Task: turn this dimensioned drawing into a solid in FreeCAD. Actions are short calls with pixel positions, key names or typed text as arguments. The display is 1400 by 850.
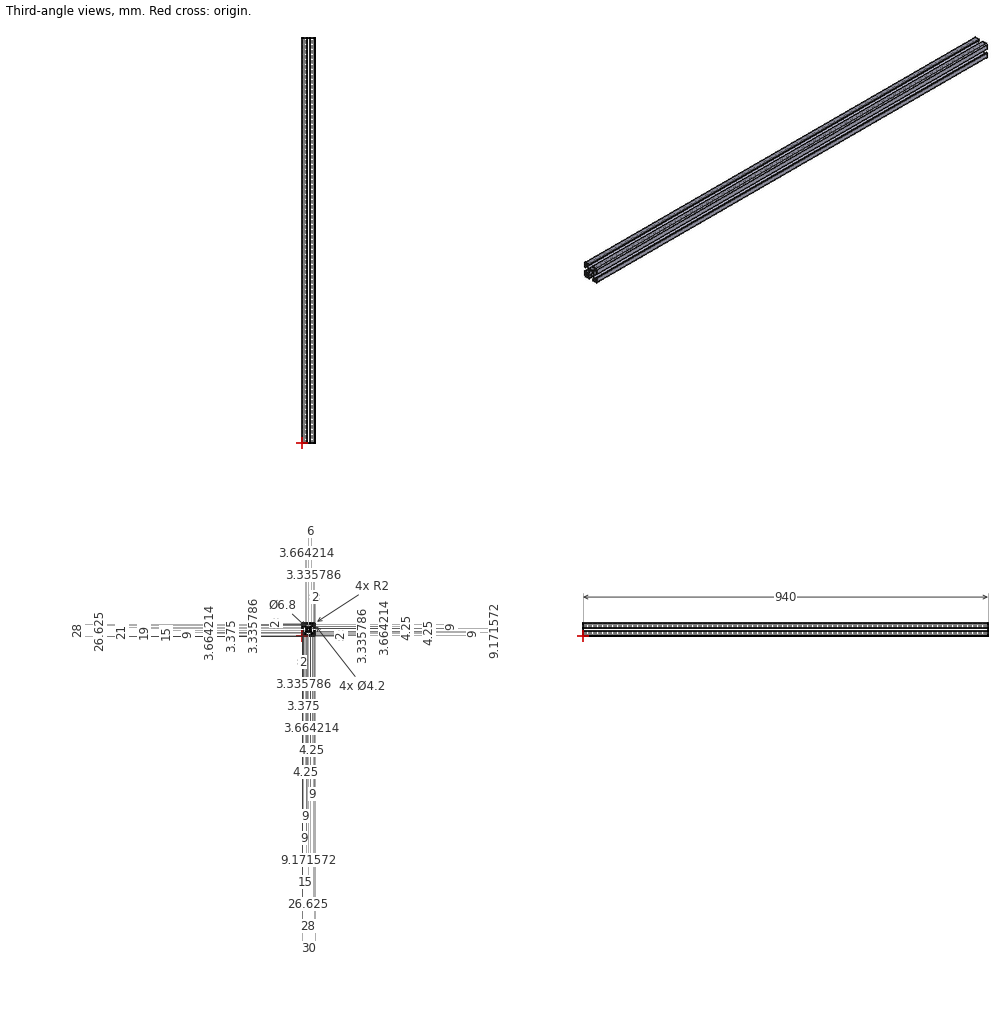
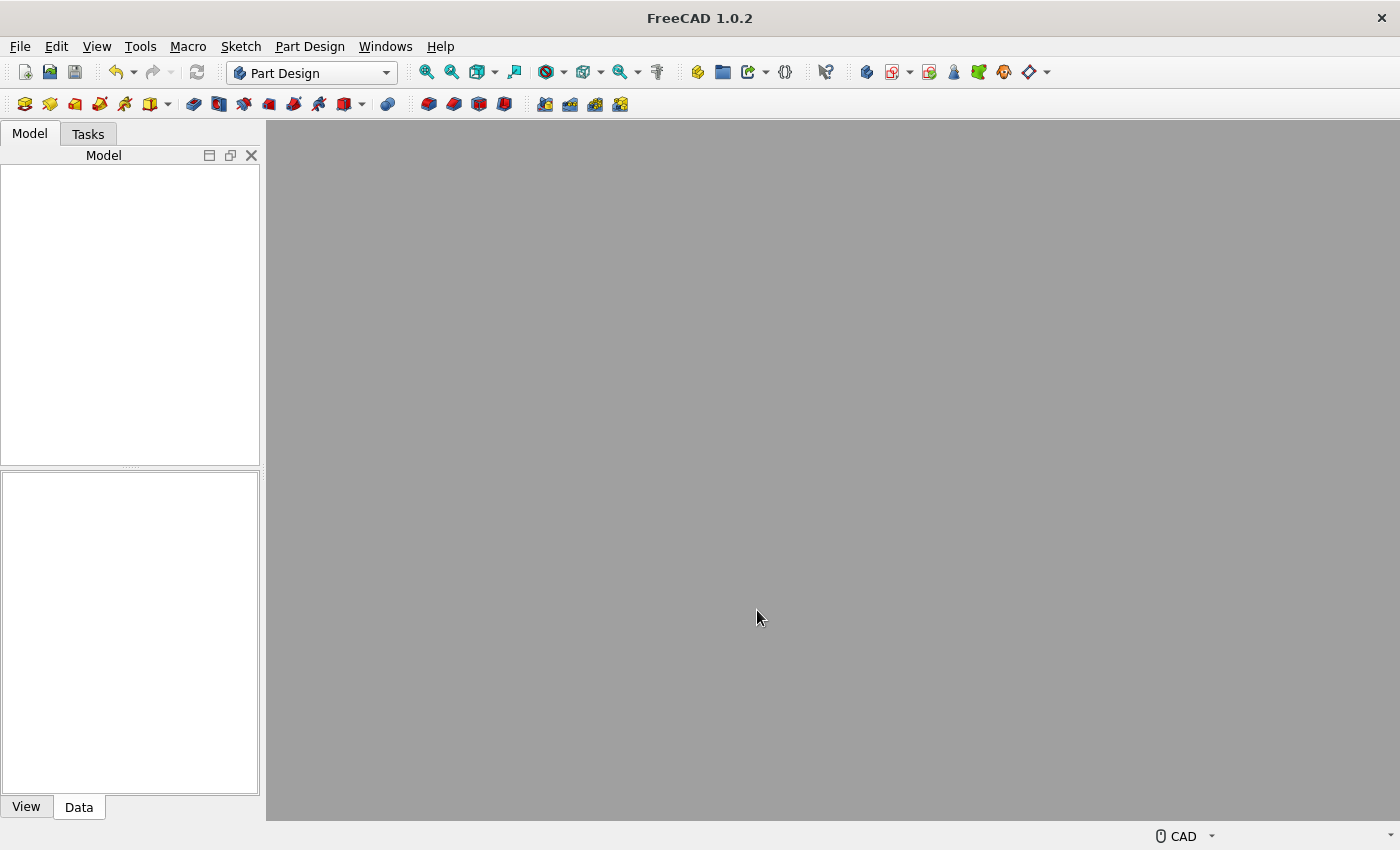
click(25, 72)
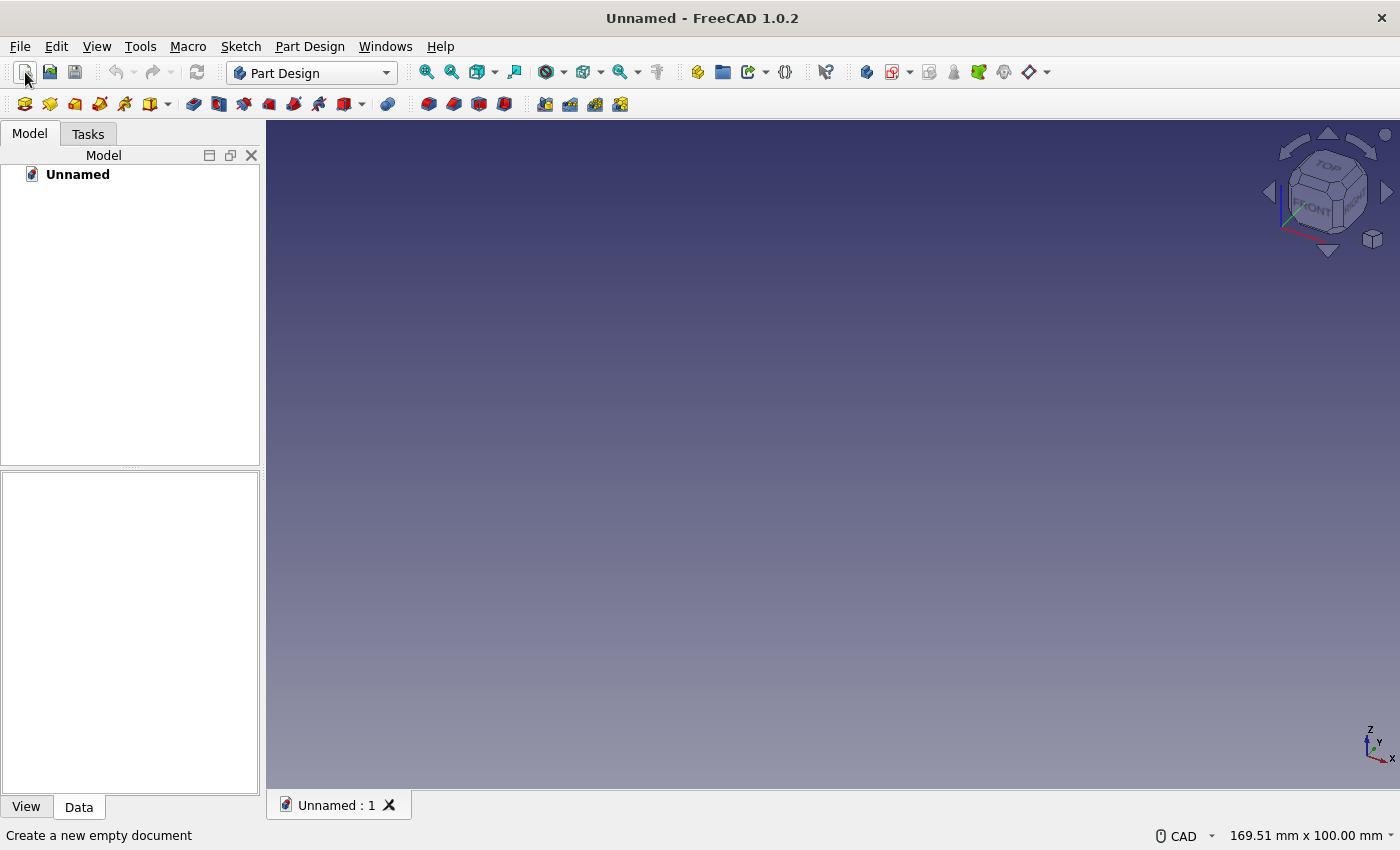
click(892, 72)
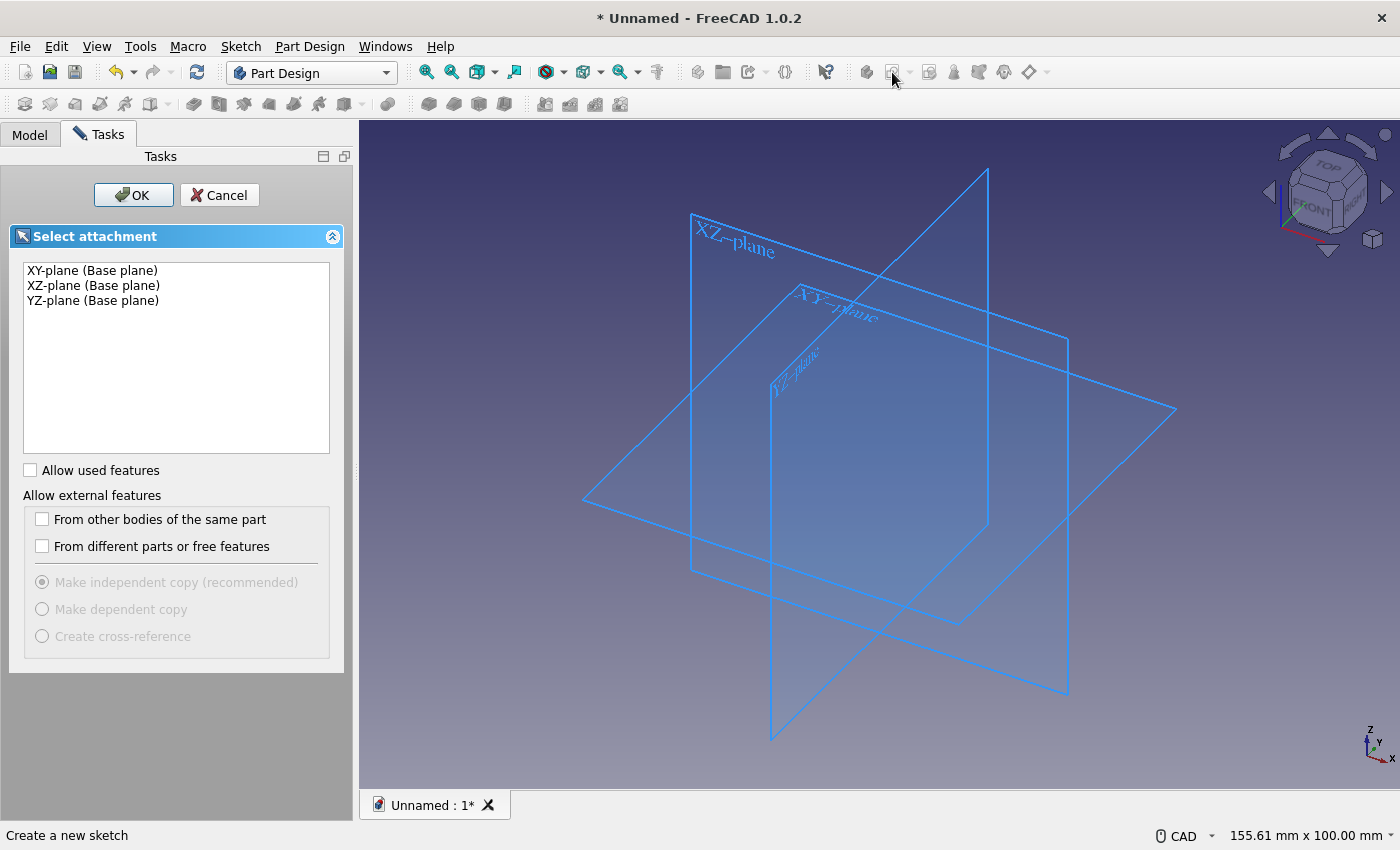
click(84, 286)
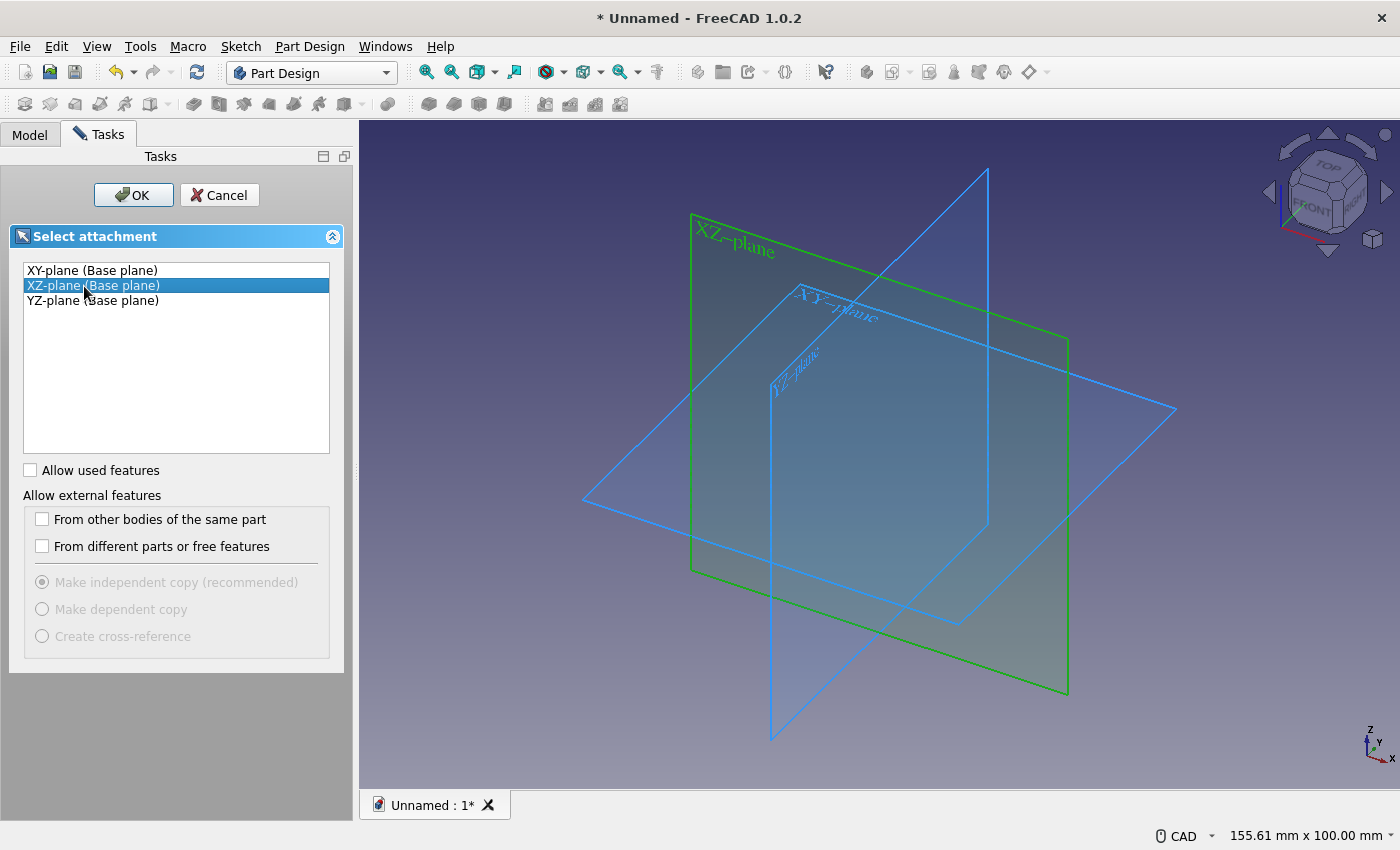
click(134, 195)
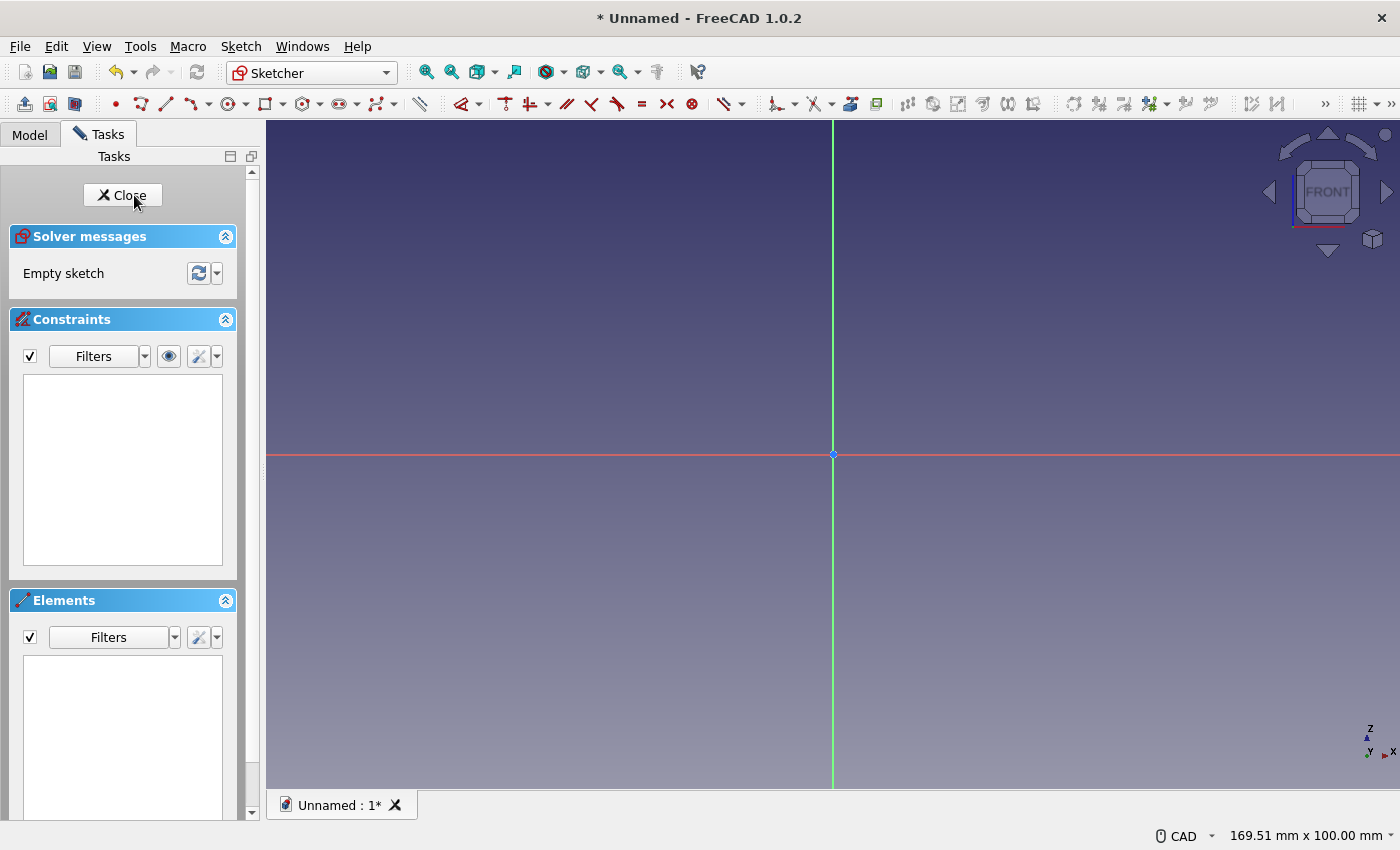
scroll(1071, 272, up, 4)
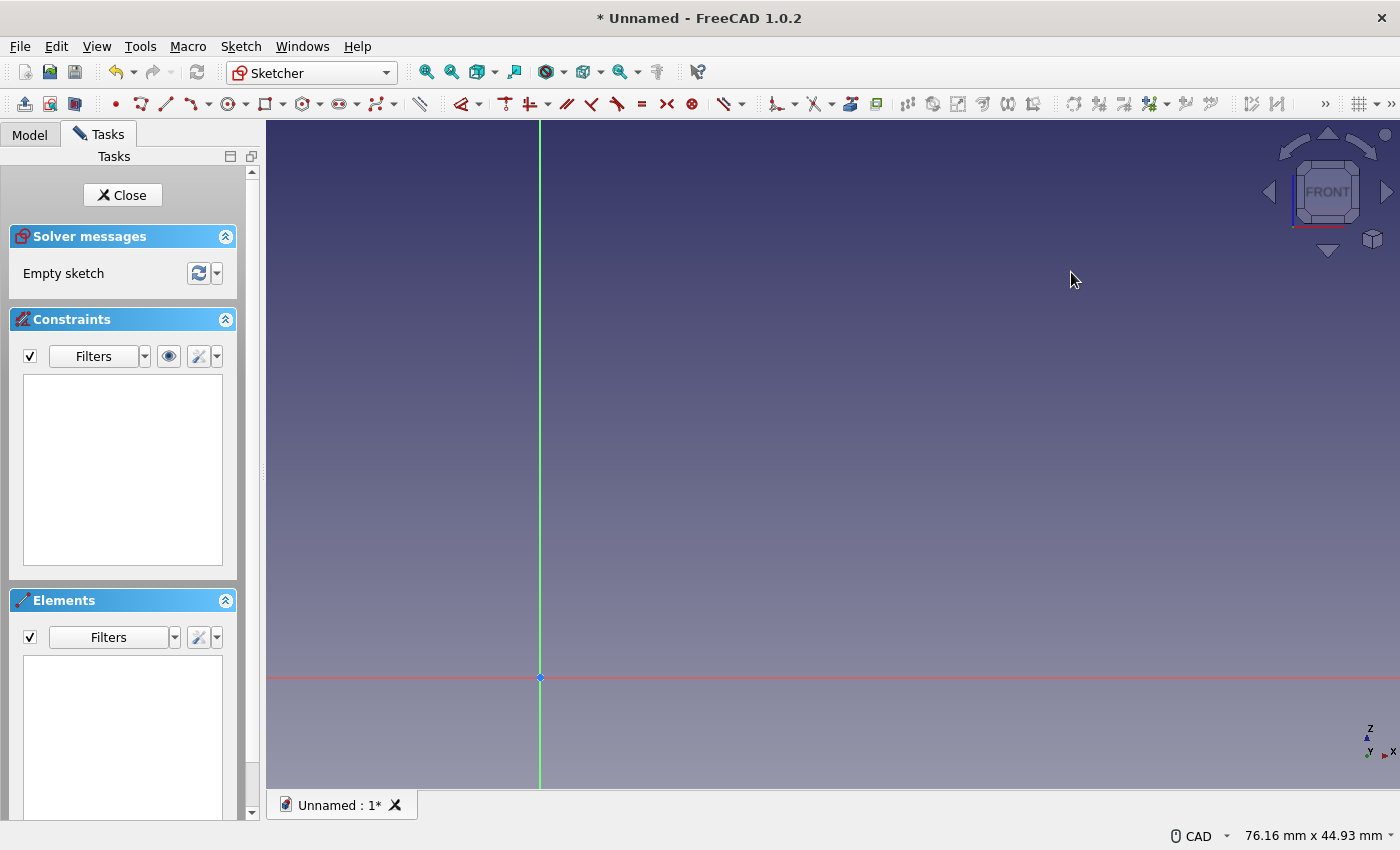
click(141, 104)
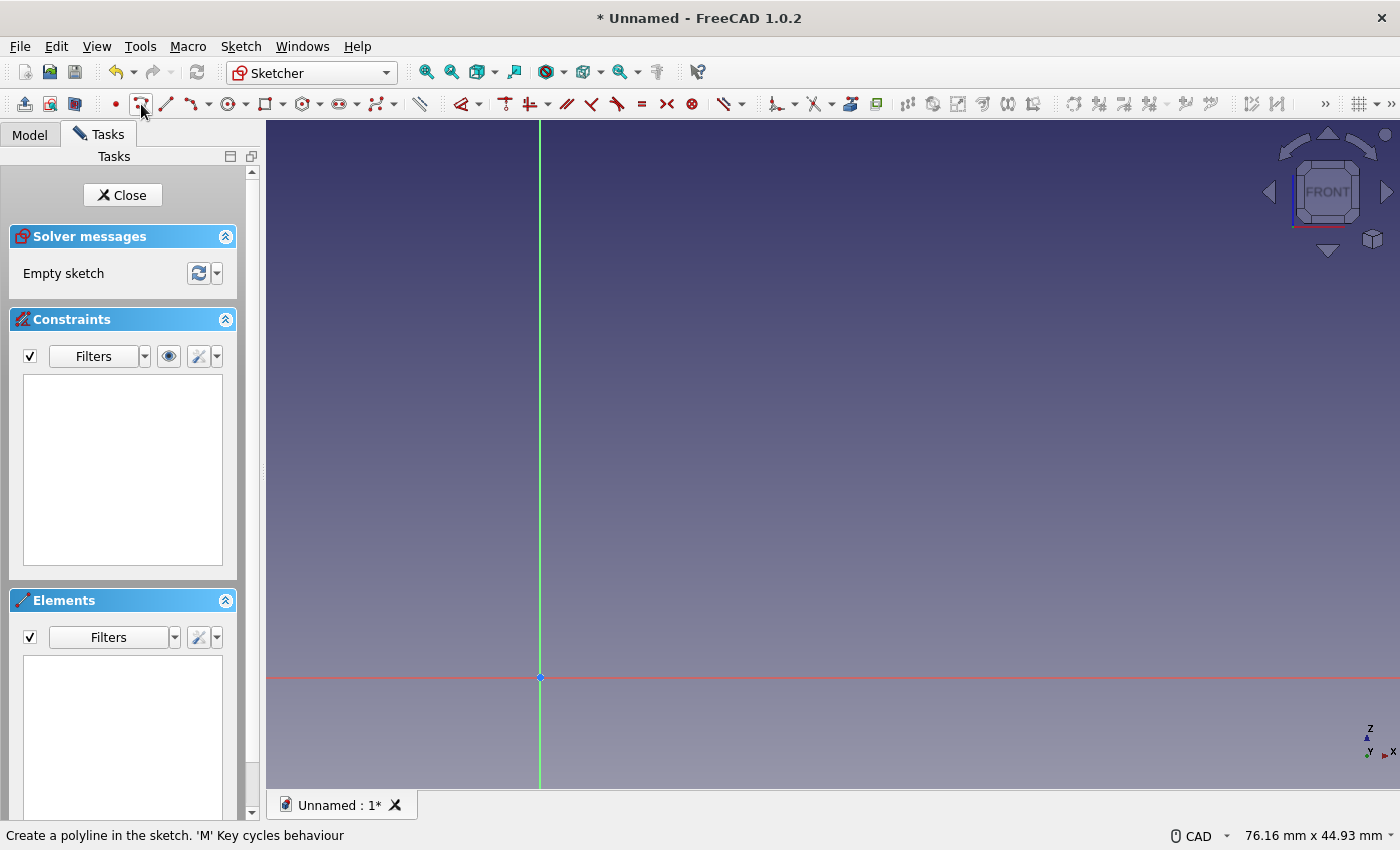
click(987, 261)
click(987, 395)
click(957, 395)
click(957, 332)
click(908, 332)
click(853, 386)
click(853, 523)
click(908, 577)
click(957, 577)
click(957, 514)
click(987, 514)
click(987, 648)
right_click(987, 648)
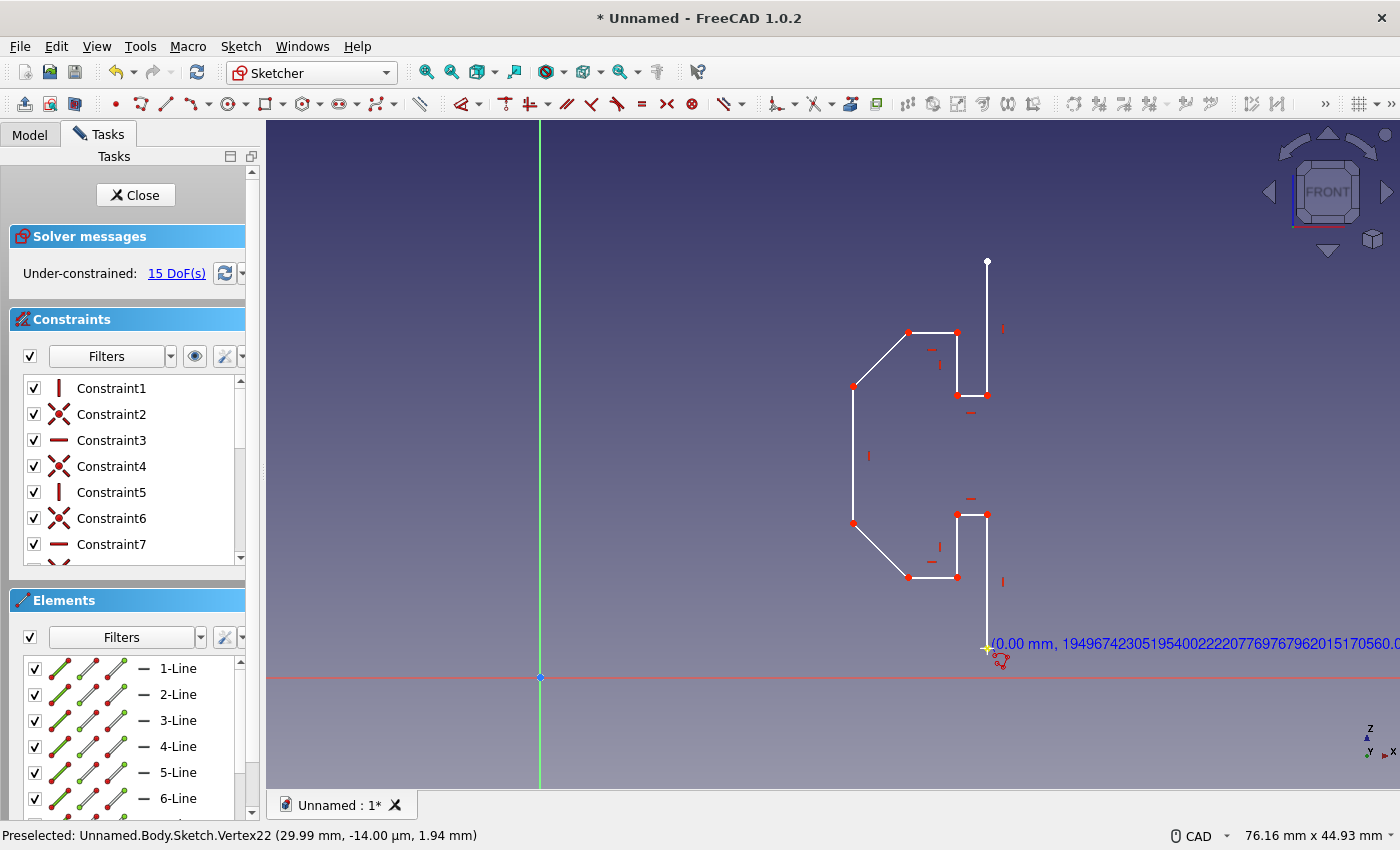
click(957, 678)
click(823, 669)
click(823, 648)
click(887, 648)
click(887, 598)
click(832, 544)
click(696, 544)
click(641, 598)
click(641, 648)
click(704, 648)
click(704, 678)
click(570, 669)
right_click(570, 669)